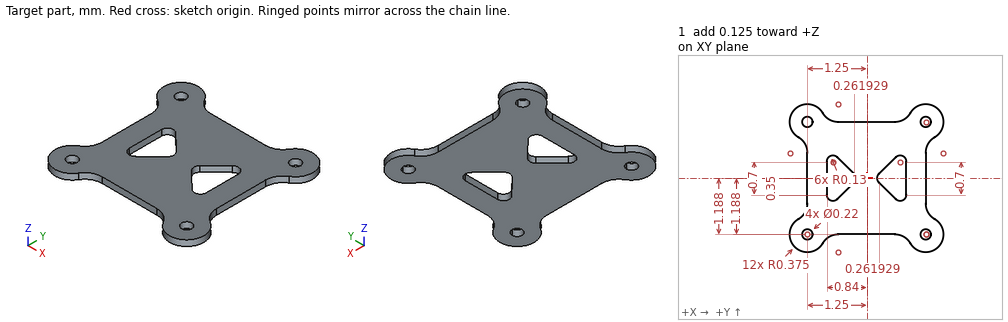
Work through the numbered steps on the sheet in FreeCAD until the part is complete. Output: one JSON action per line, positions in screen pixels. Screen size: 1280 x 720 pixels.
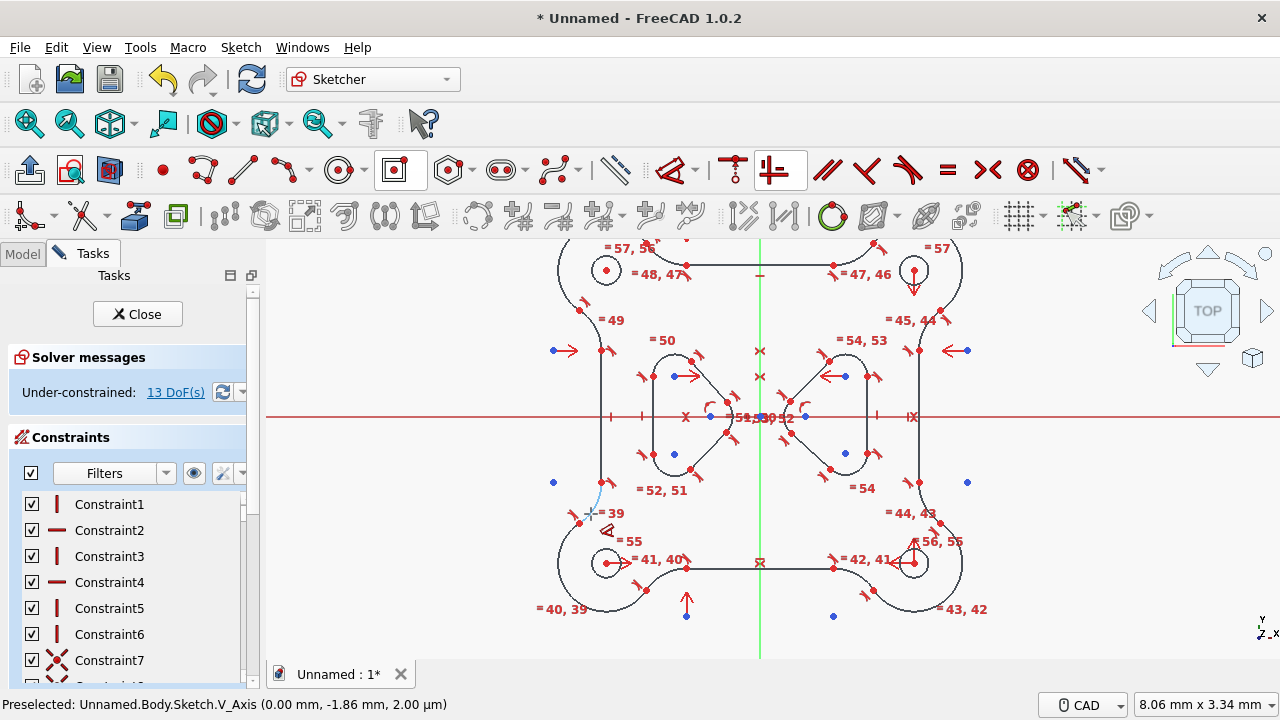
{"action": "left_click", "coordinate": [590, 514]}
{"action": "left_click", "coordinate": [614, 535]}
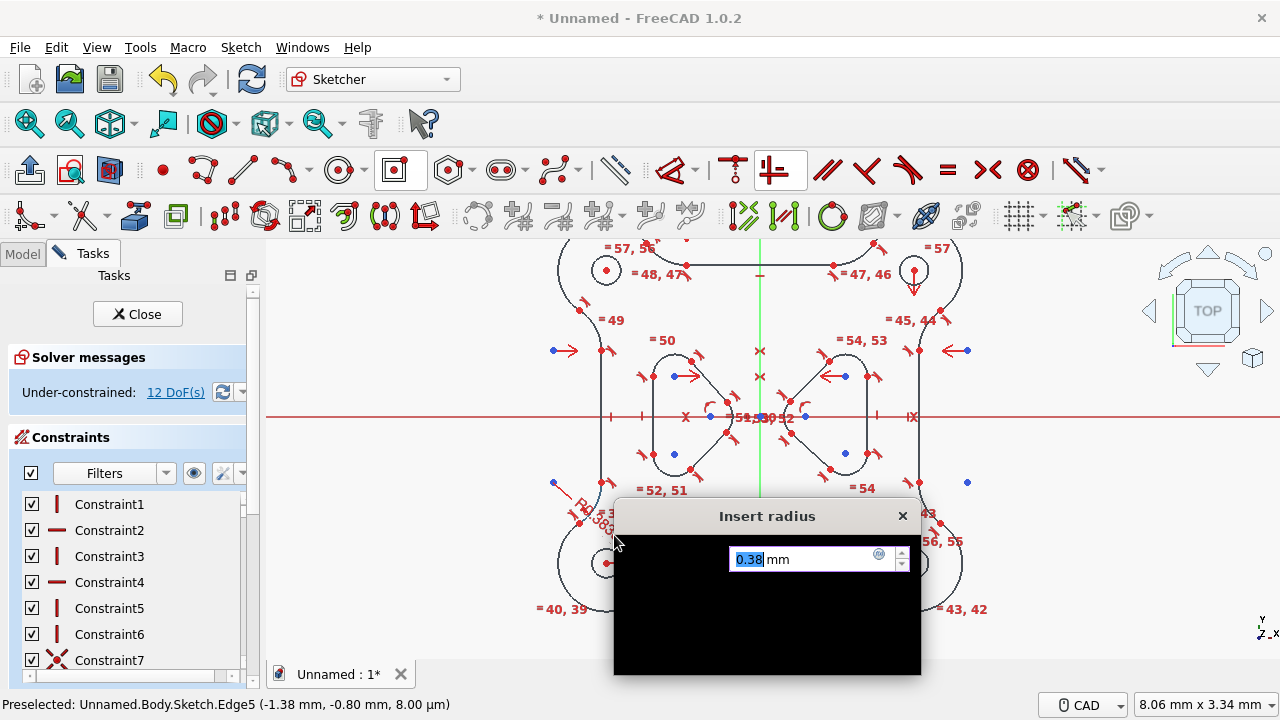
{"action": "type", "text": "0.375"}
{"action": "key", "text": "Return"}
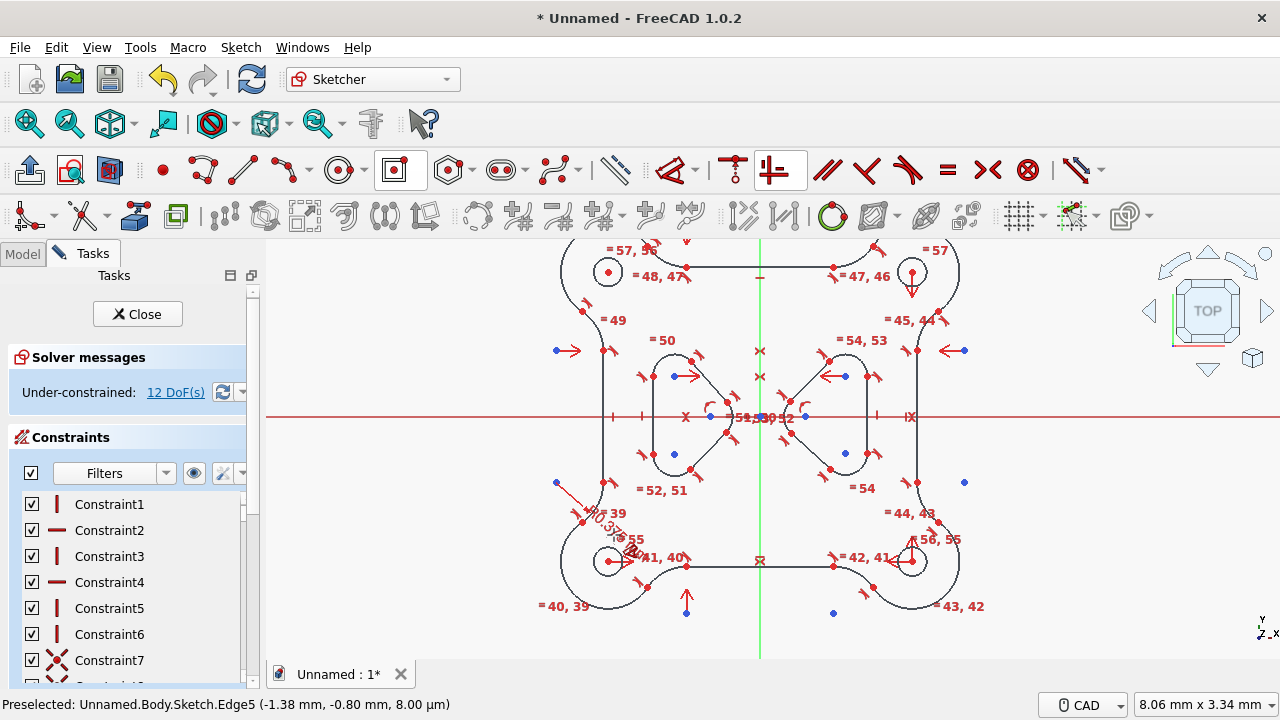
{"action": "scroll", "coordinate": [678, 355], "scroll_direction": "up", "scroll_amount": 5}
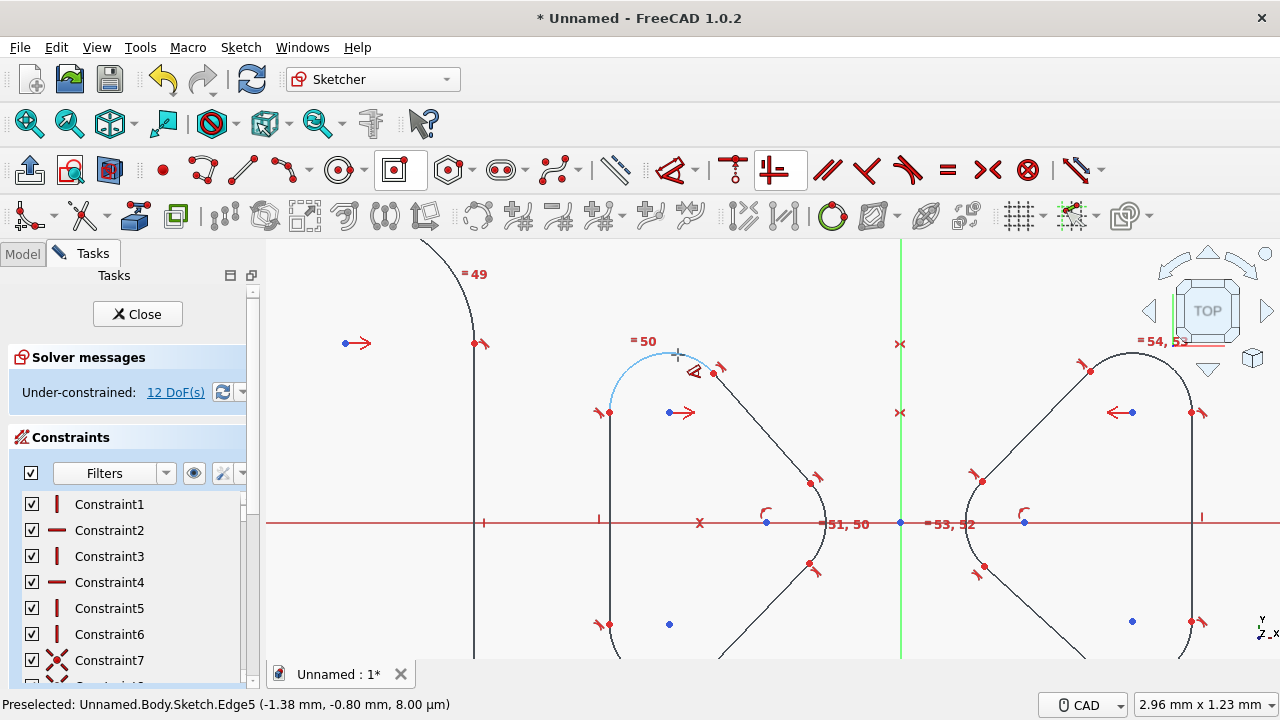
{"action": "left_click", "coordinate": [676, 354]}
{"action": "left_click", "coordinate": [680, 322]}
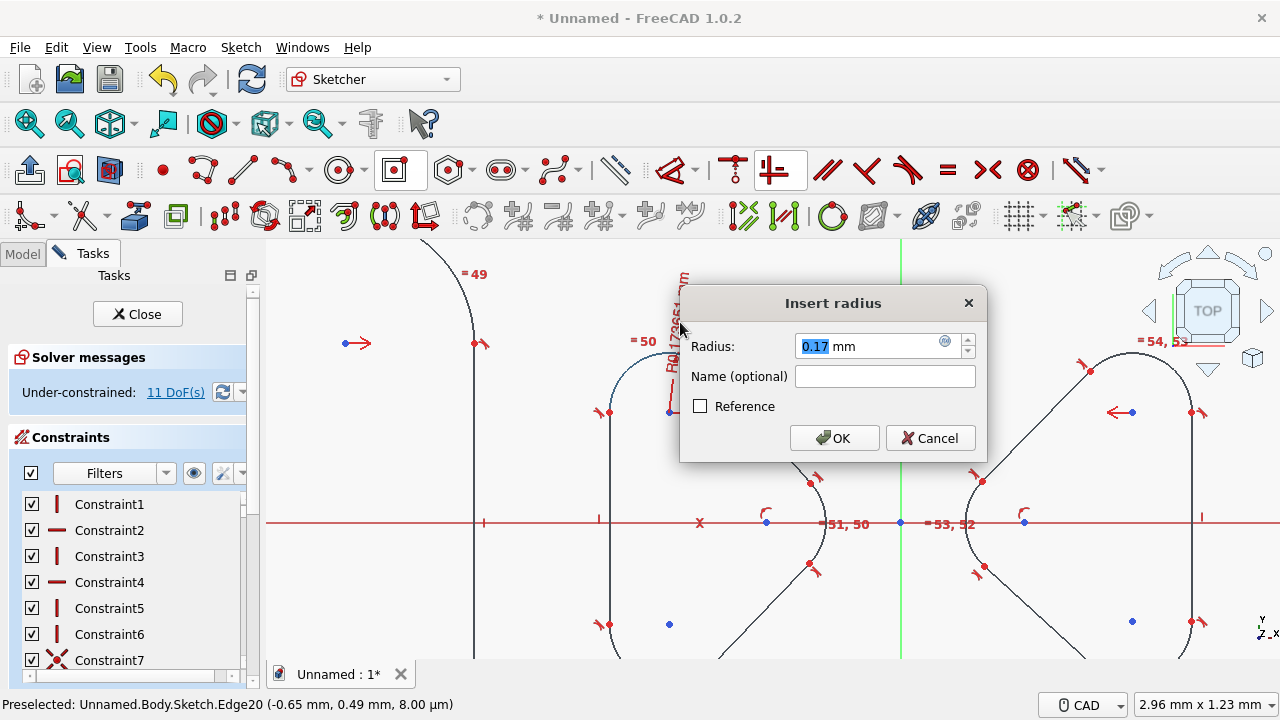
{"action": "type", "text": "0.13"}
{"action": "key", "text": "Return"}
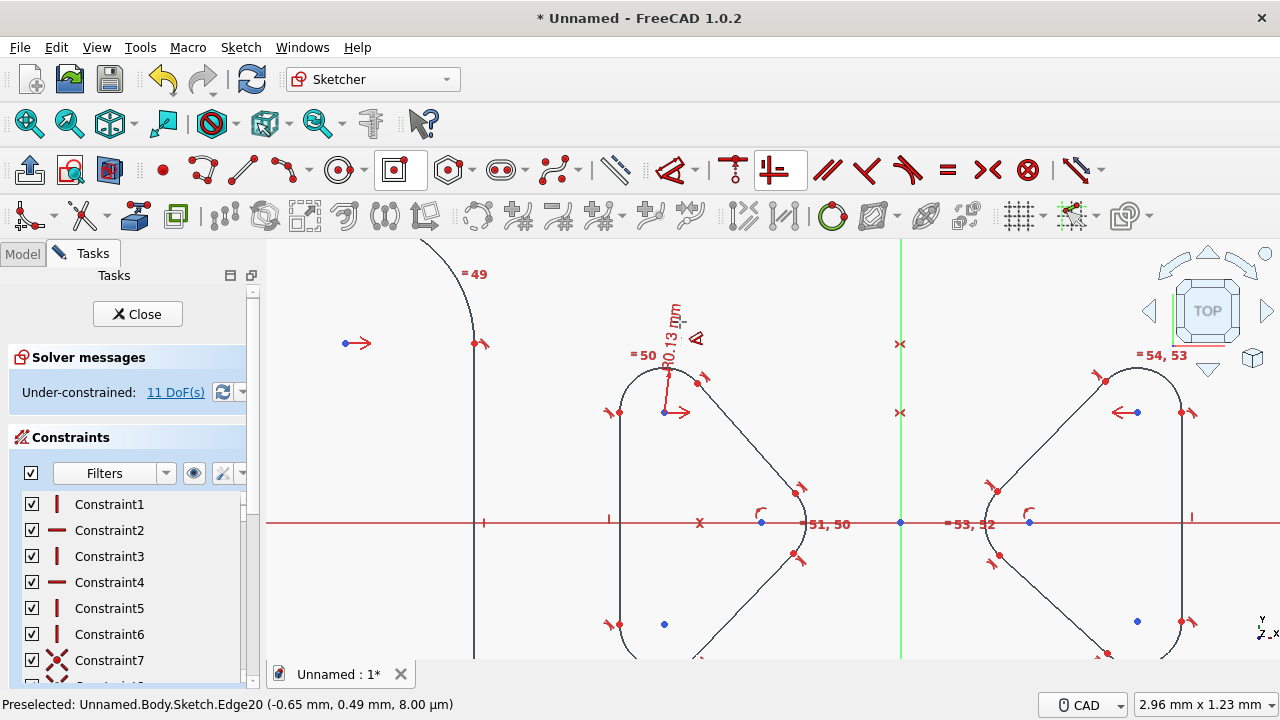
{"action": "scroll", "coordinate": [640, 425], "scroll_direction": "down", "scroll_amount": 7}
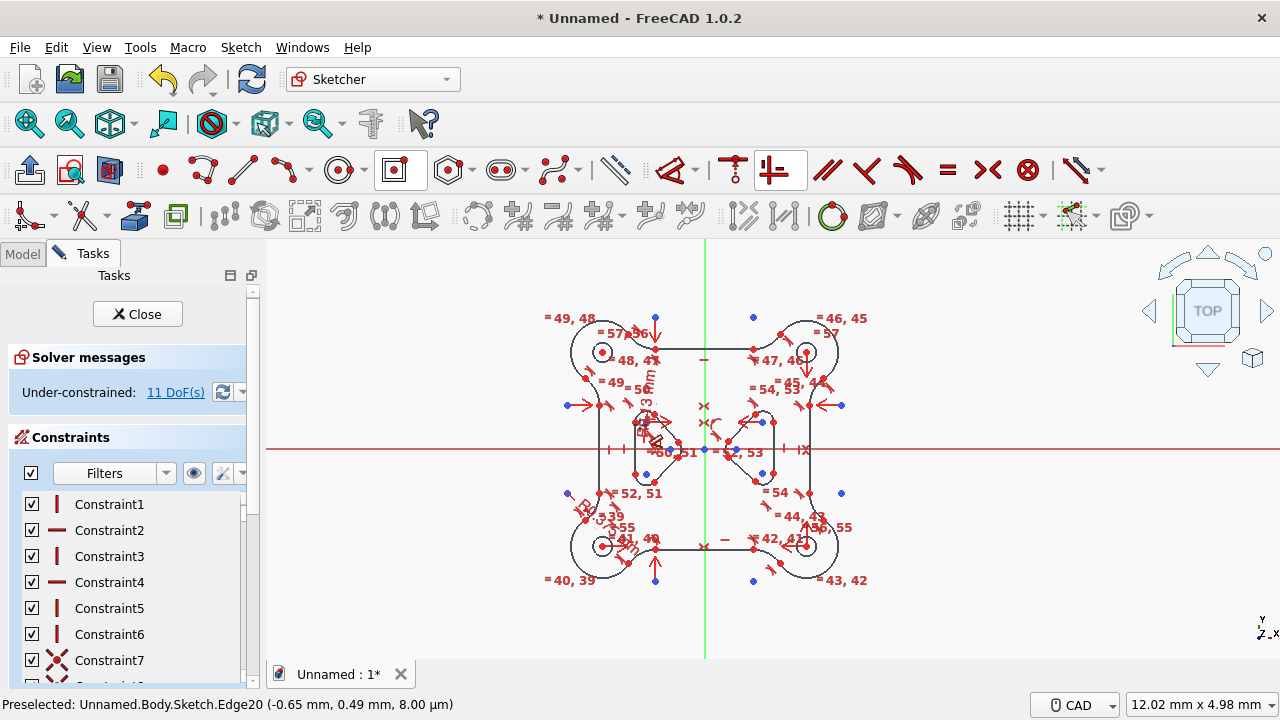
{"action": "scroll", "coordinate": [609, 540], "scroll_direction": "up", "scroll_amount": 4}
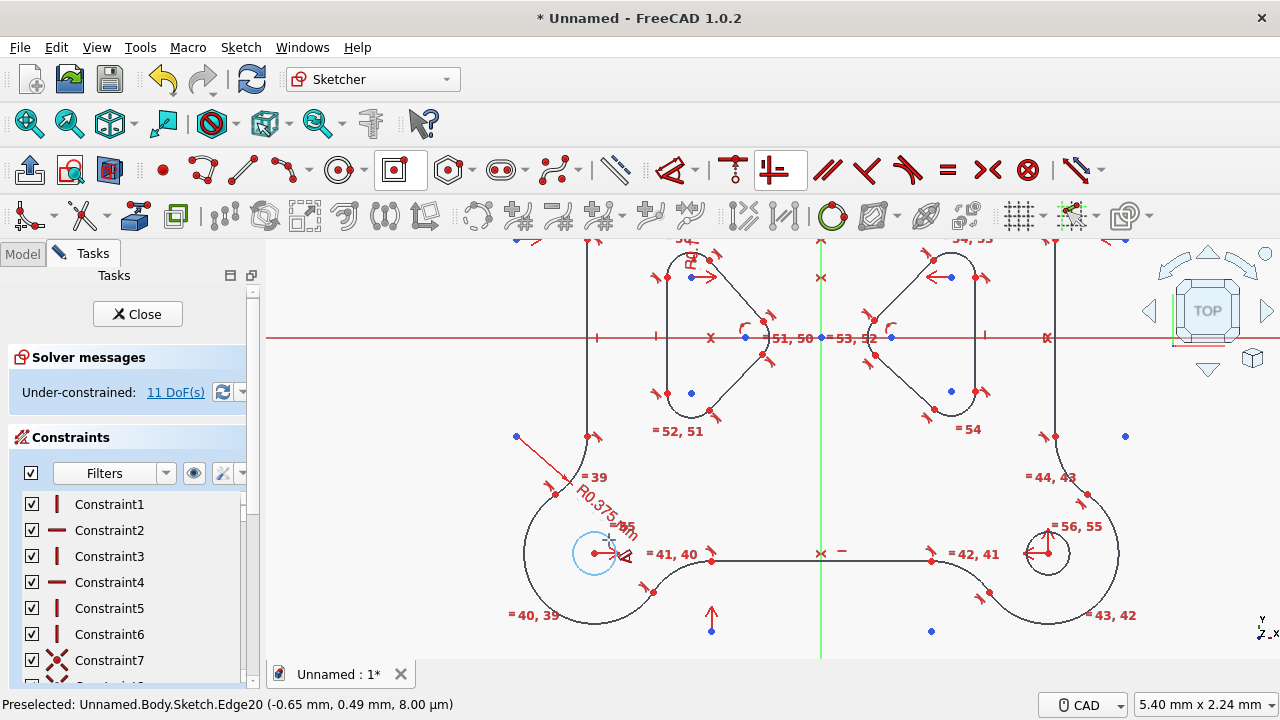
{"action": "left_click", "coordinate": [609, 538]}
{"action": "left_click", "coordinate": [645, 537]}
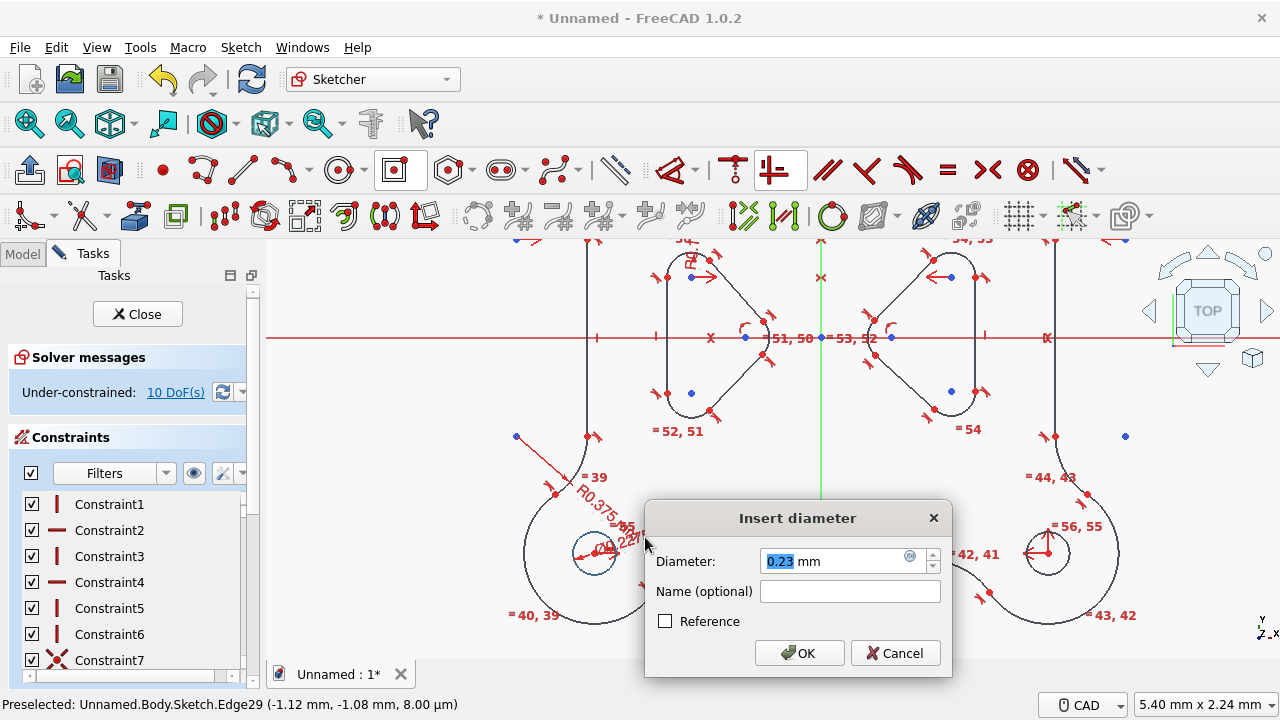
{"action": "type", "text": "0.22"}
{"action": "key", "text": "Return"}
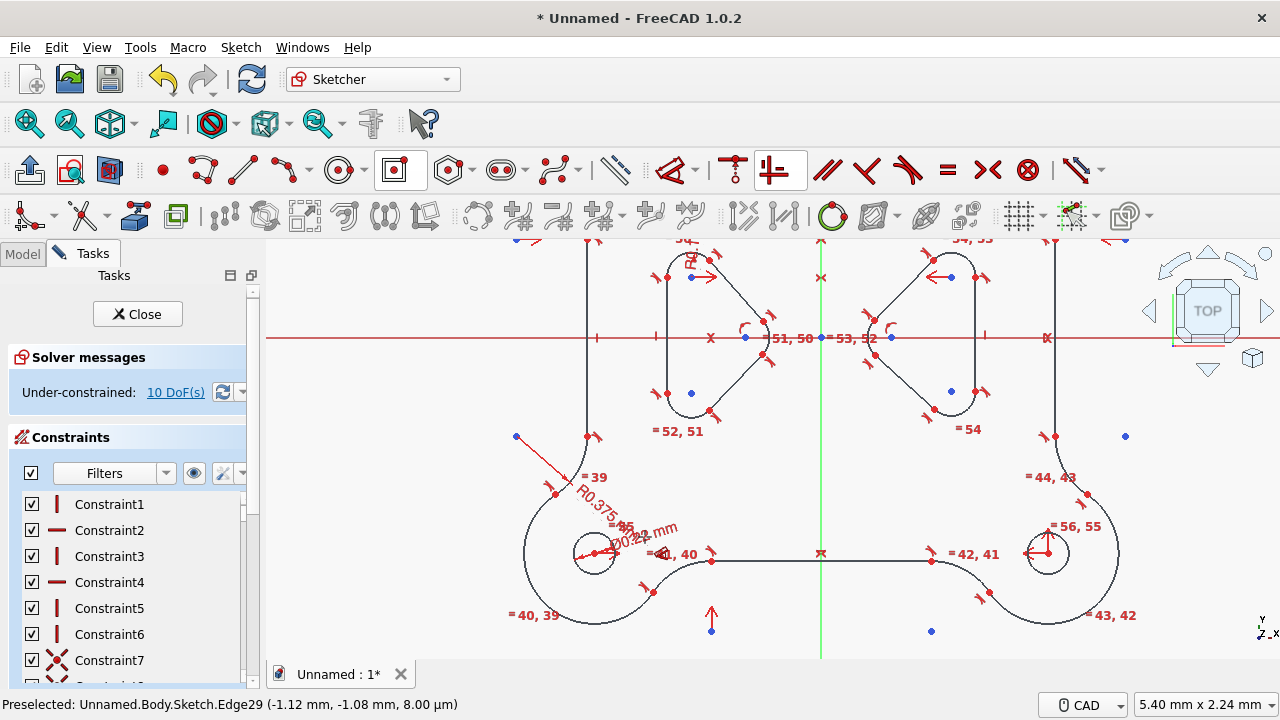
{"action": "left_click", "coordinate": [667, 358]}
{"action": "left_click", "coordinate": [633, 308]}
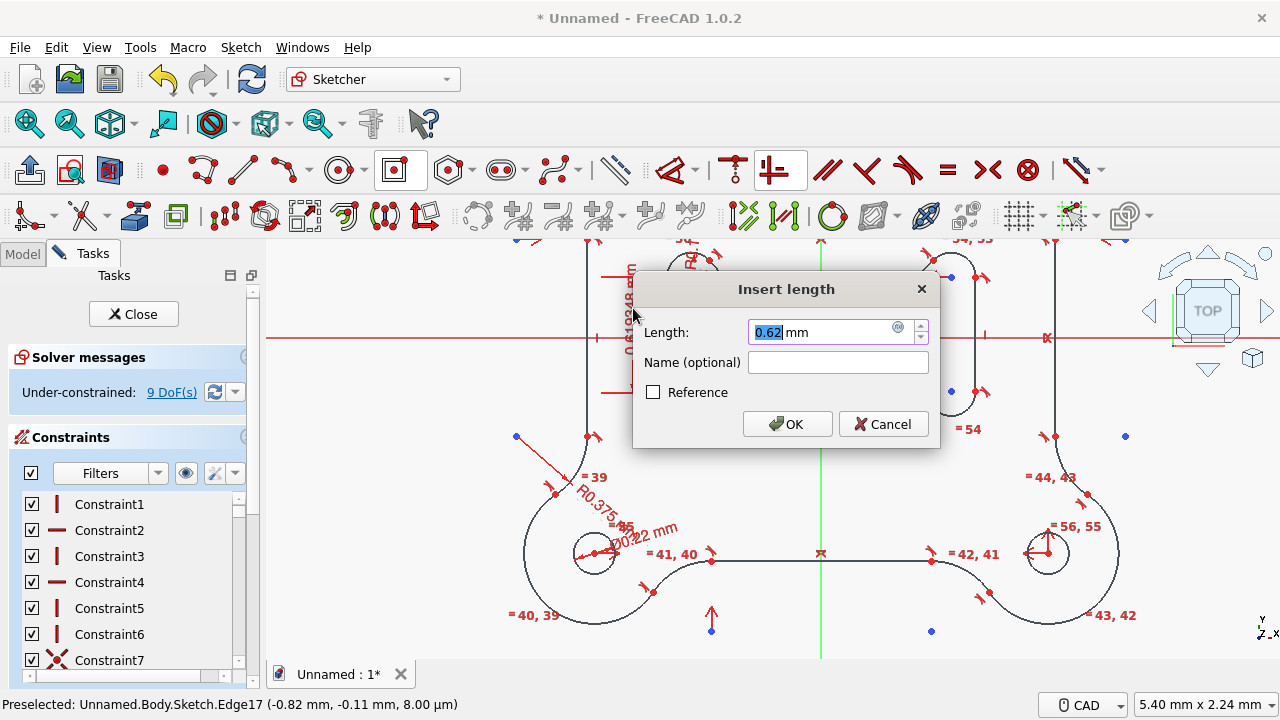
{"action": "type", "text": "0.7"}
{"action": "key", "text": "Return"}